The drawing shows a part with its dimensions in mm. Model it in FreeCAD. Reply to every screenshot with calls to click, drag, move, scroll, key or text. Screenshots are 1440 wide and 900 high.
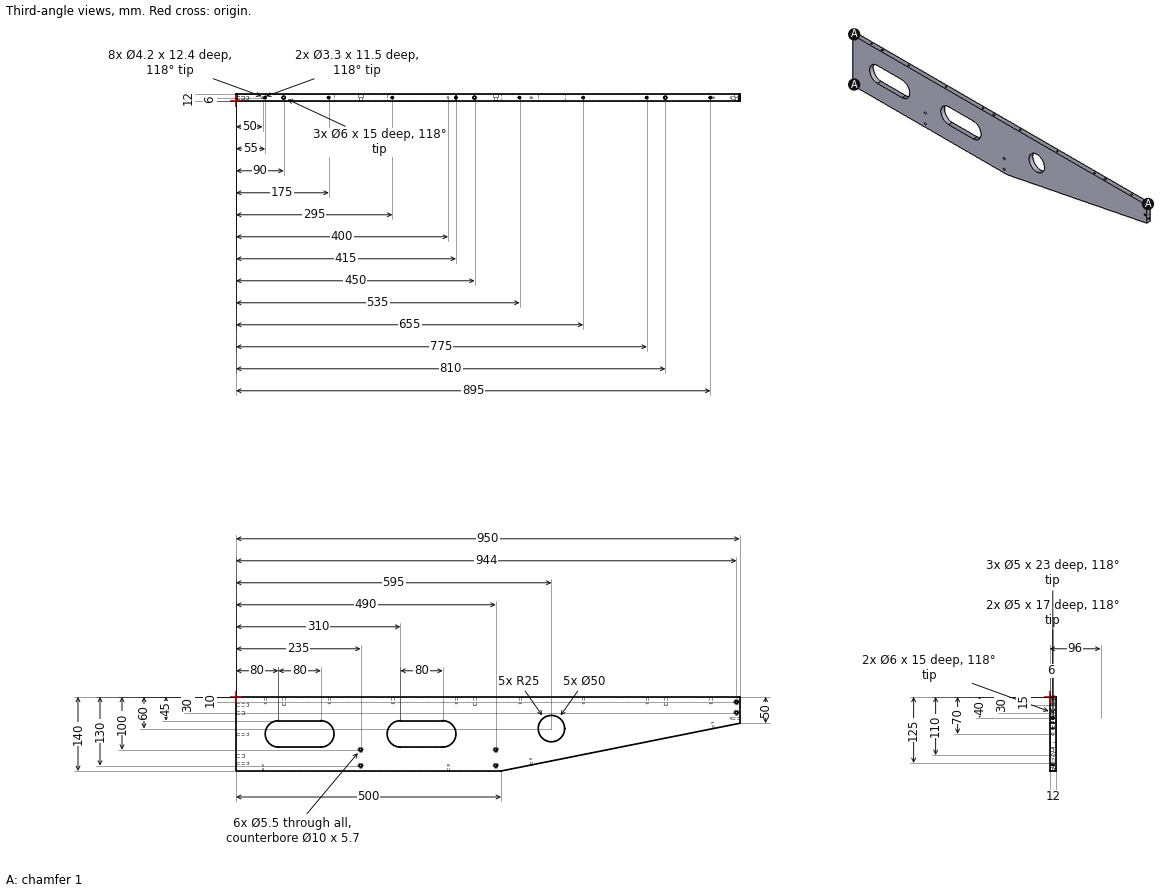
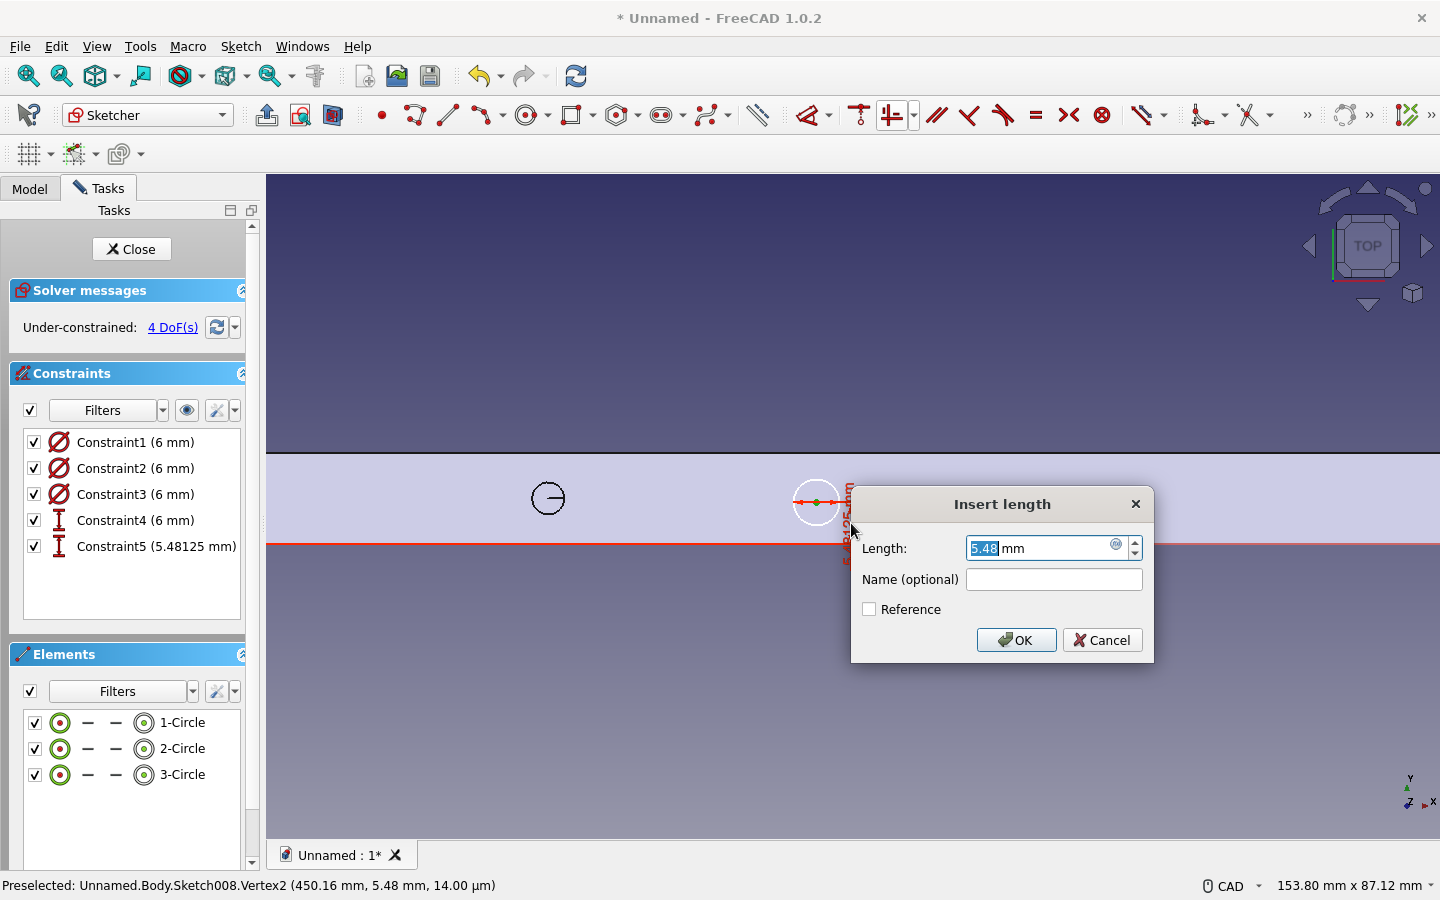
text(6)
key(Return)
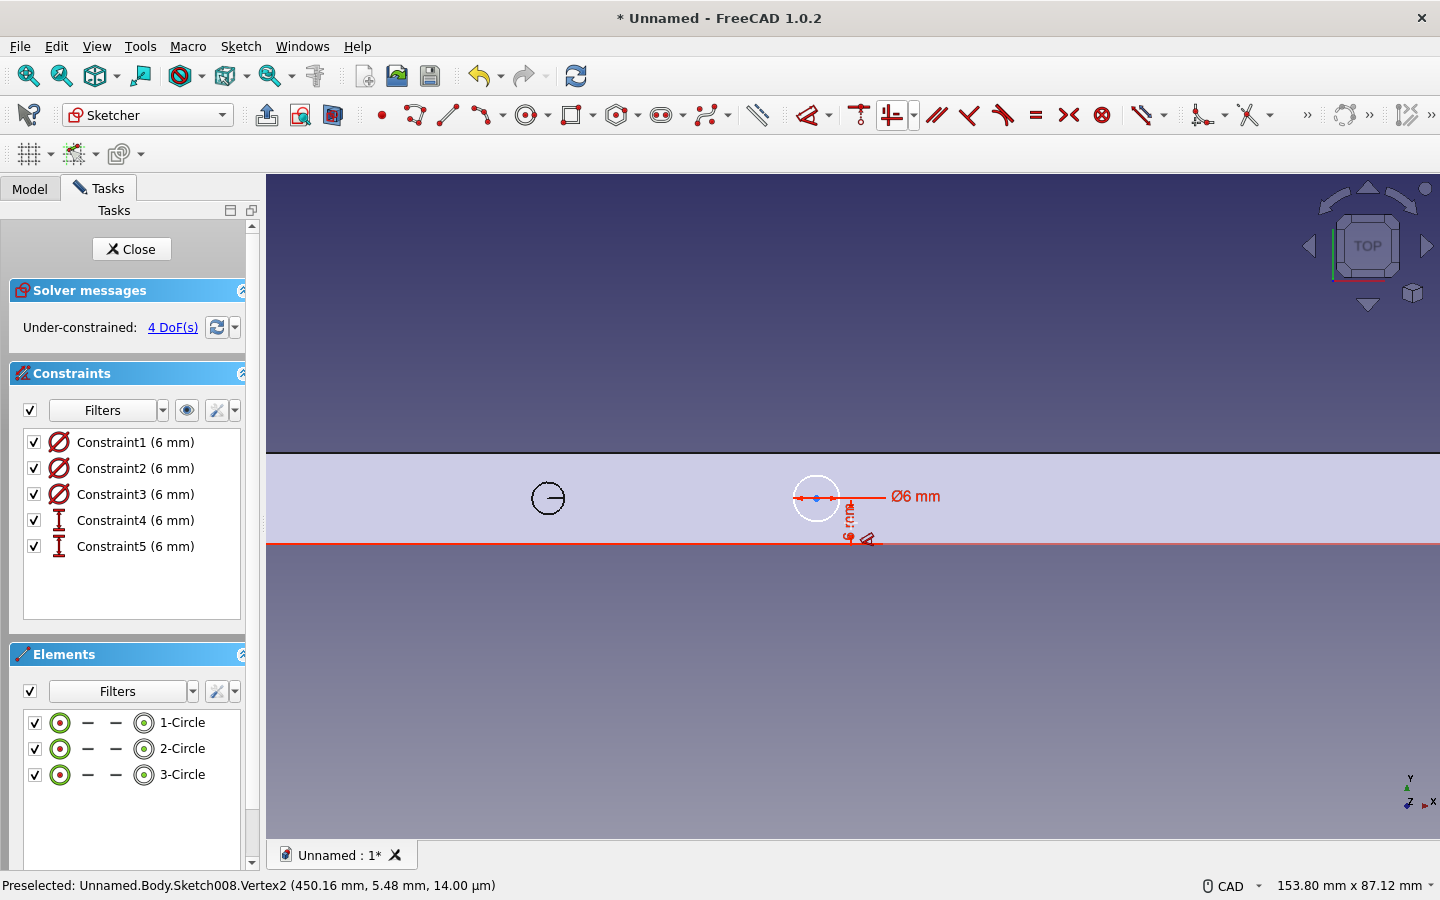
scroll(822, 506, down, 11)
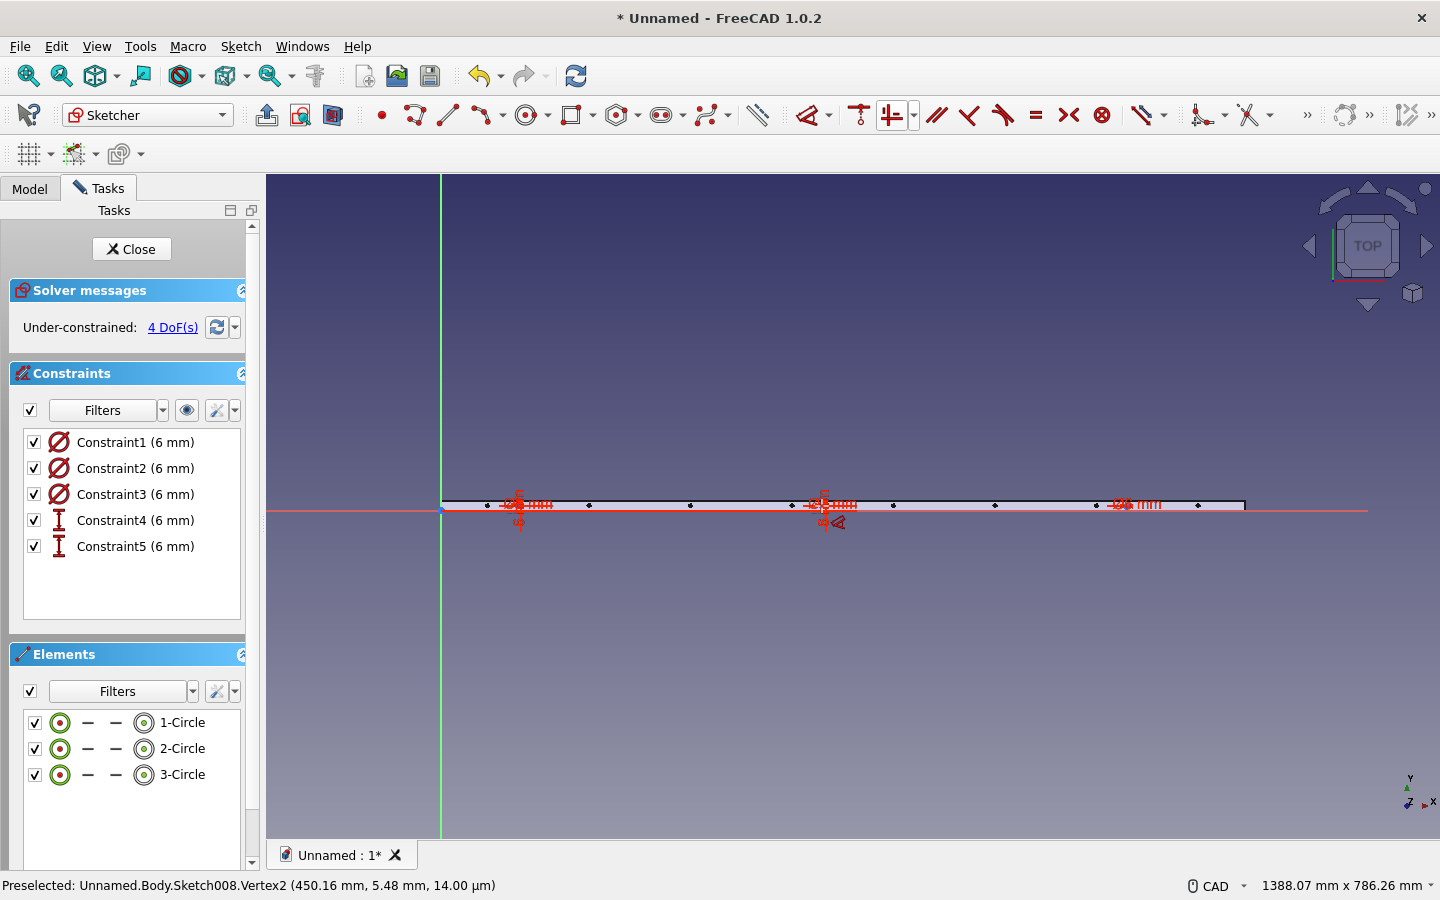
scroll(1126, 506, up, 11)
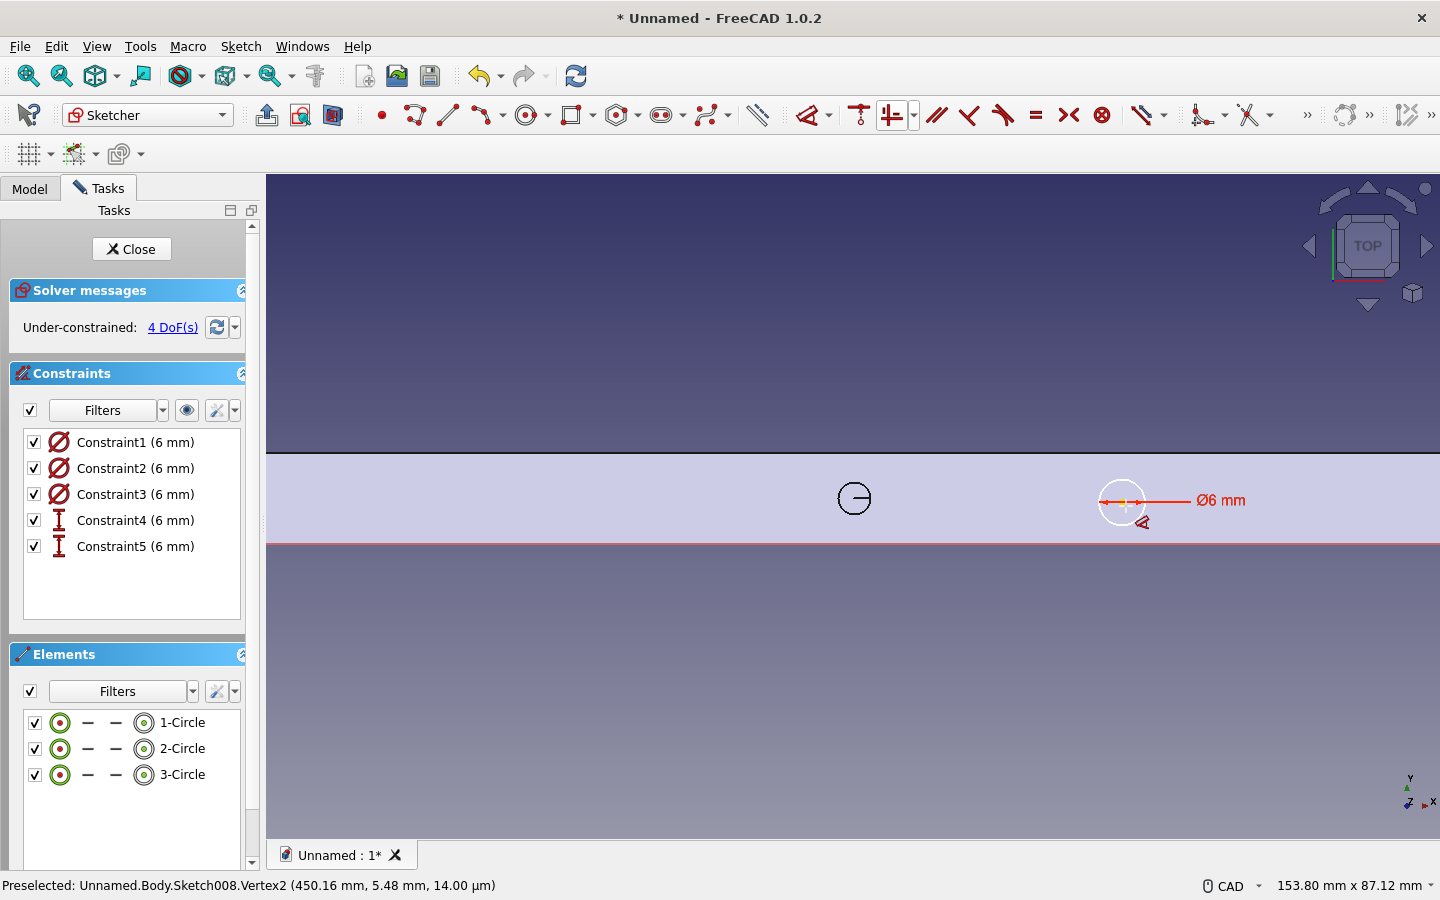
click(1122, 502)
click(1156, 523)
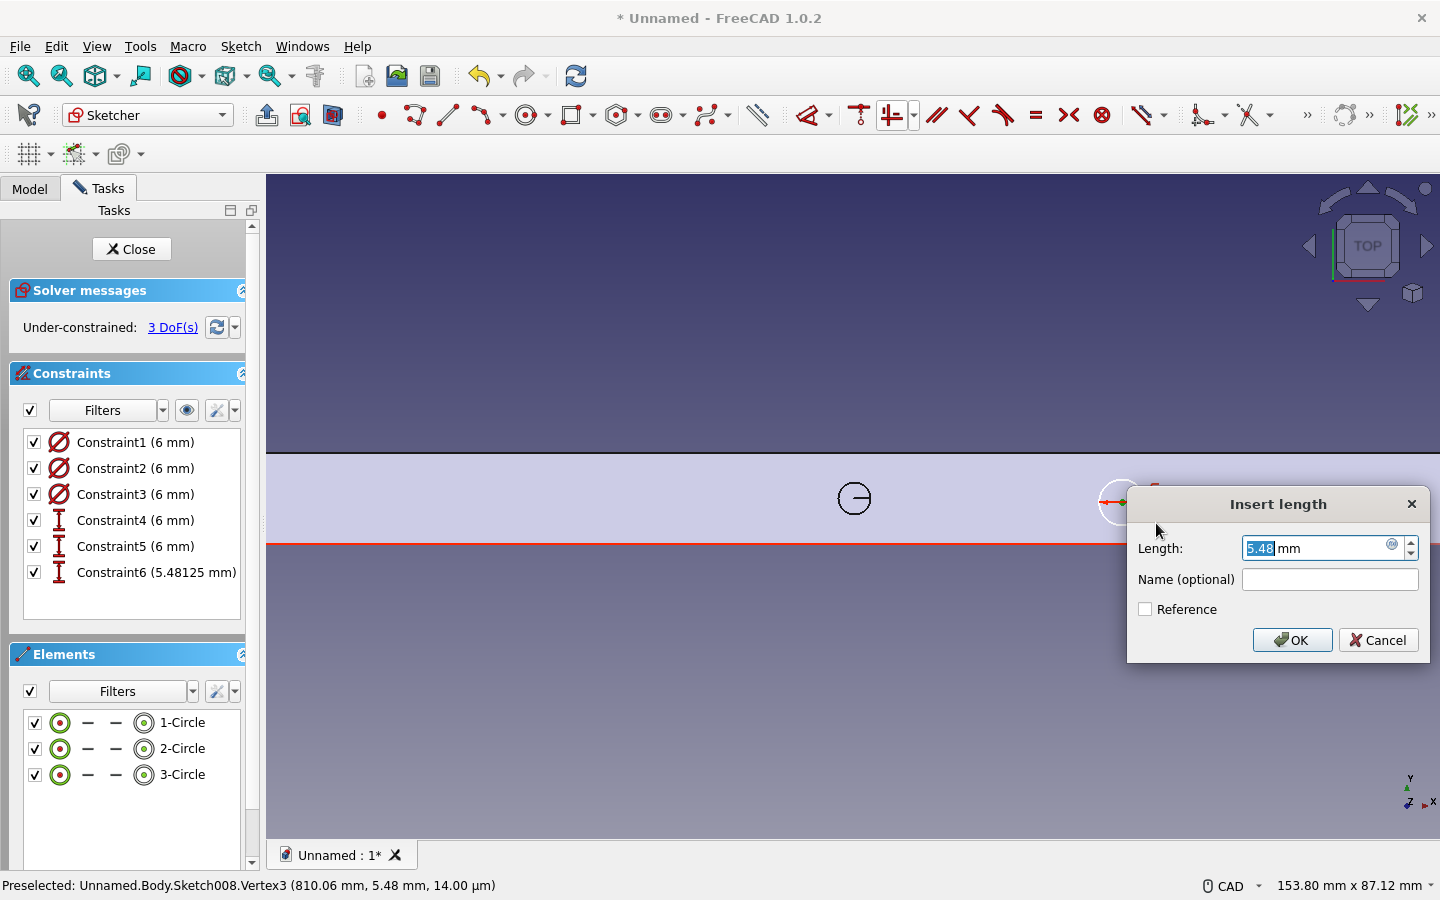
text(6)
key(Return)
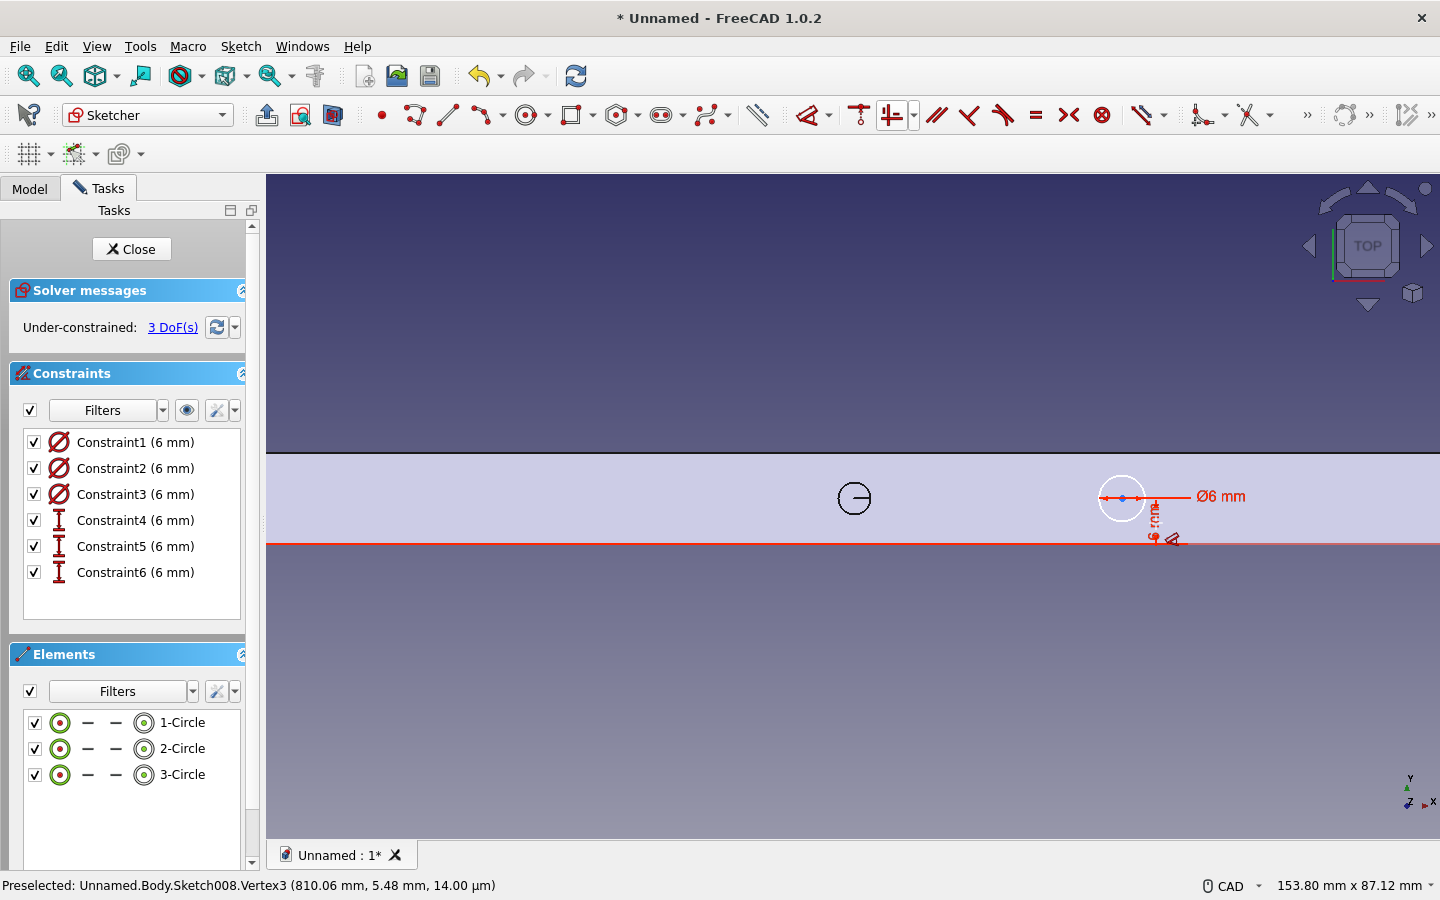
scroll(1126, 506, down, 11)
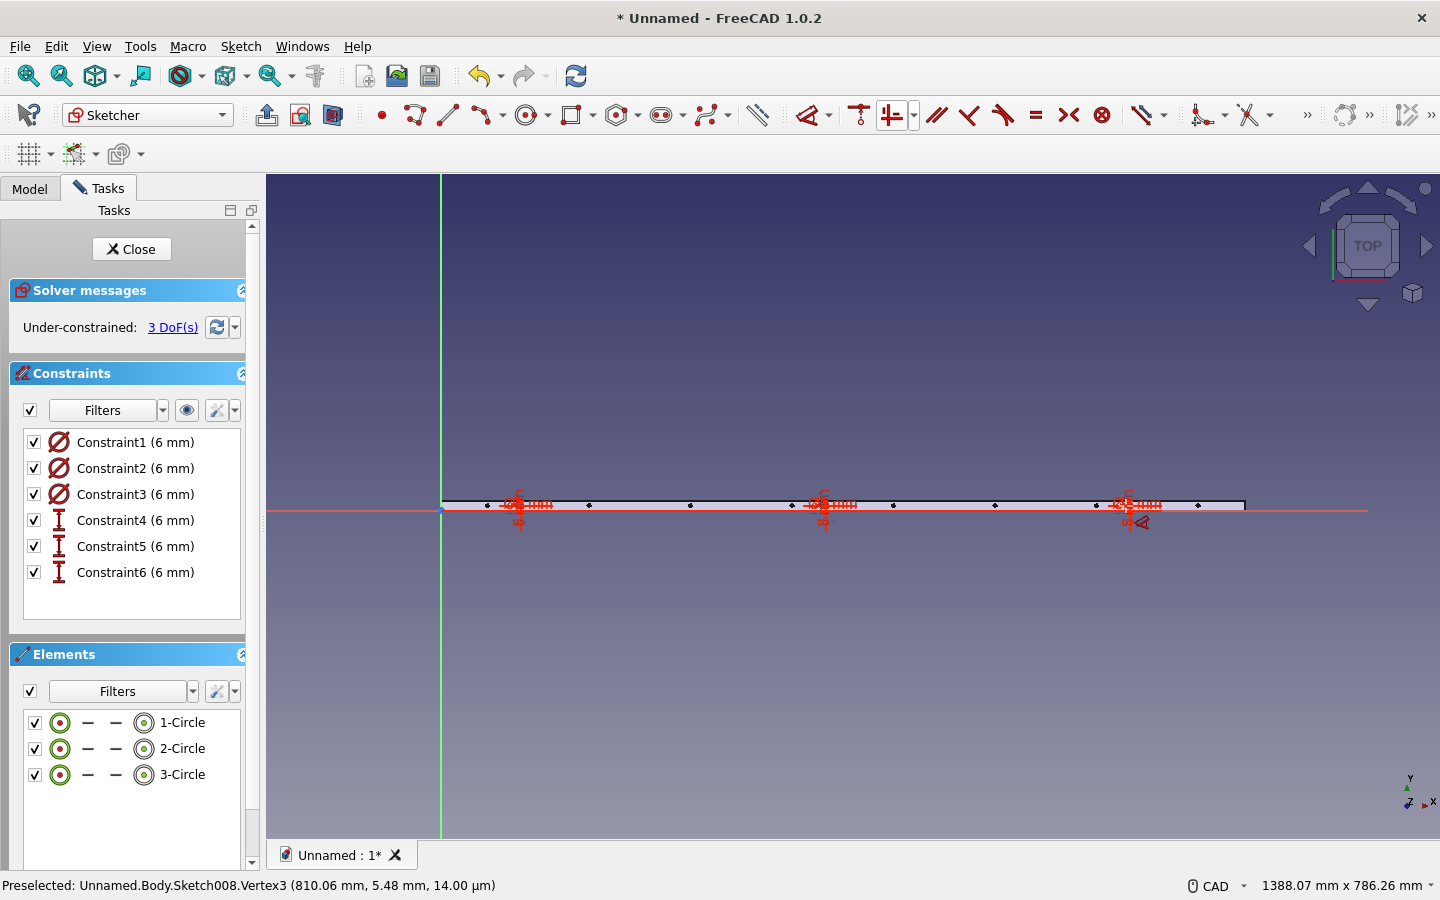
click(517, 506)
click(479, 545)